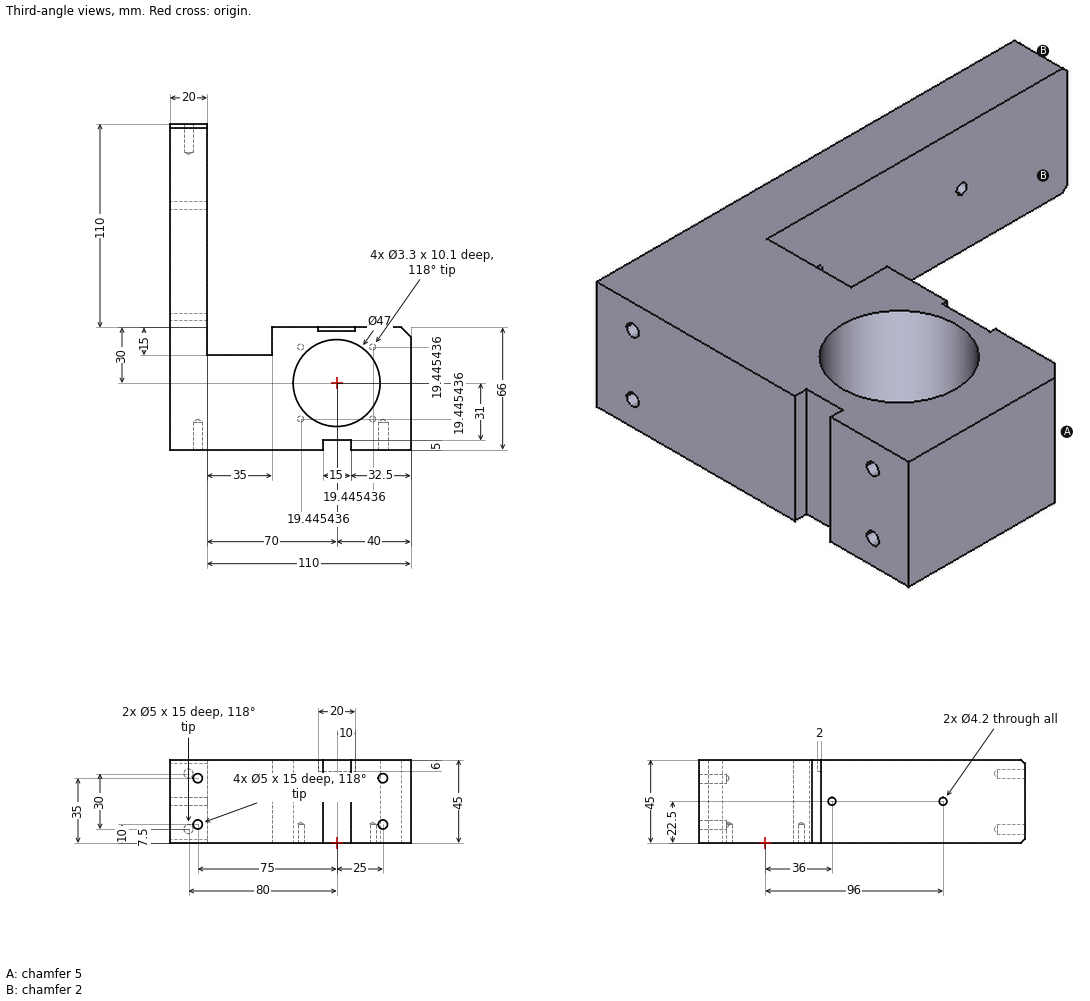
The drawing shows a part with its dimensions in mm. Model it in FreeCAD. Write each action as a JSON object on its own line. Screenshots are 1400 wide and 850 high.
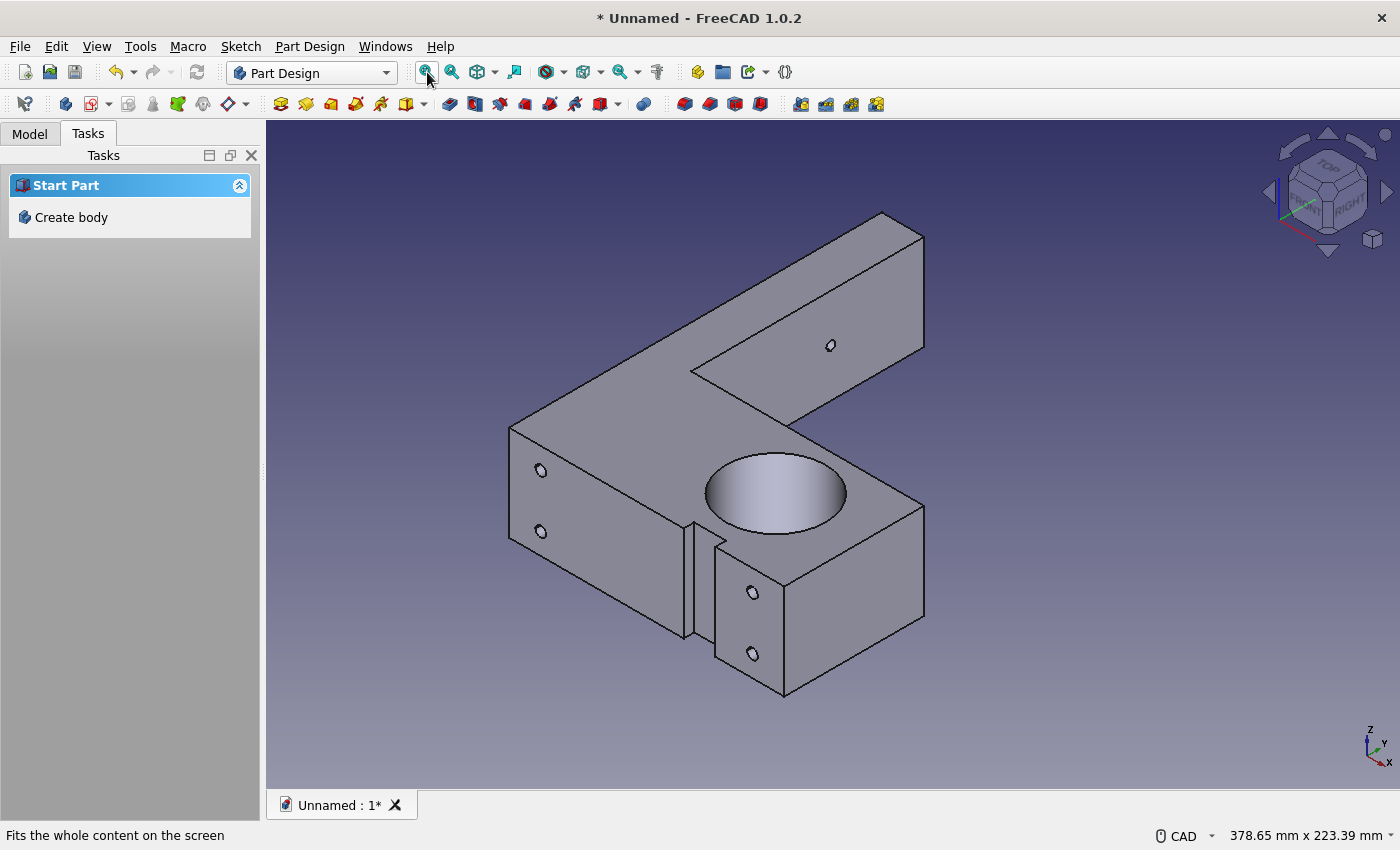
{"action": "key", "text": "2"}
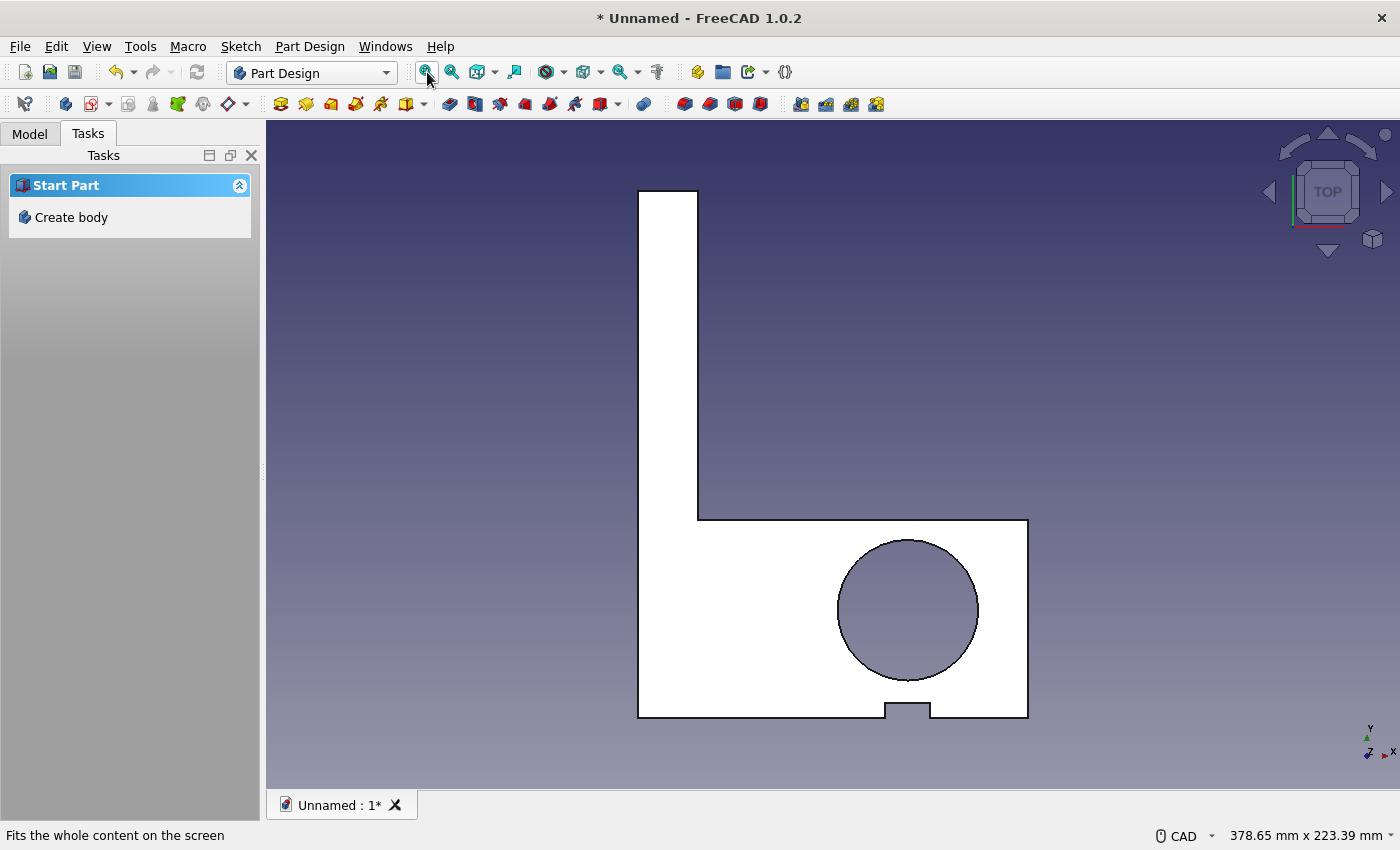
{"action": "key", "text": "1"}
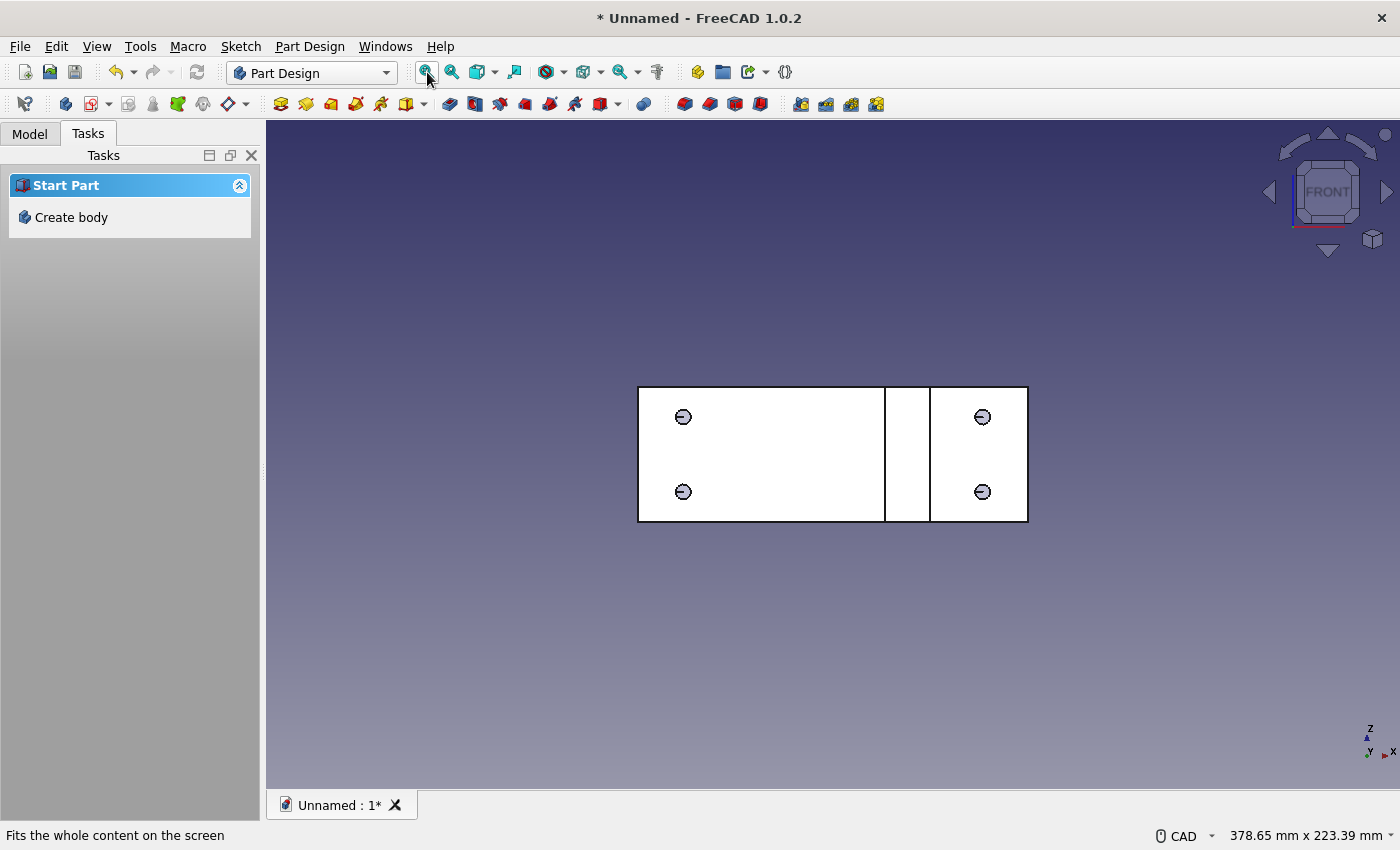
{"action": "left_click", "coordinate": [427, 72]}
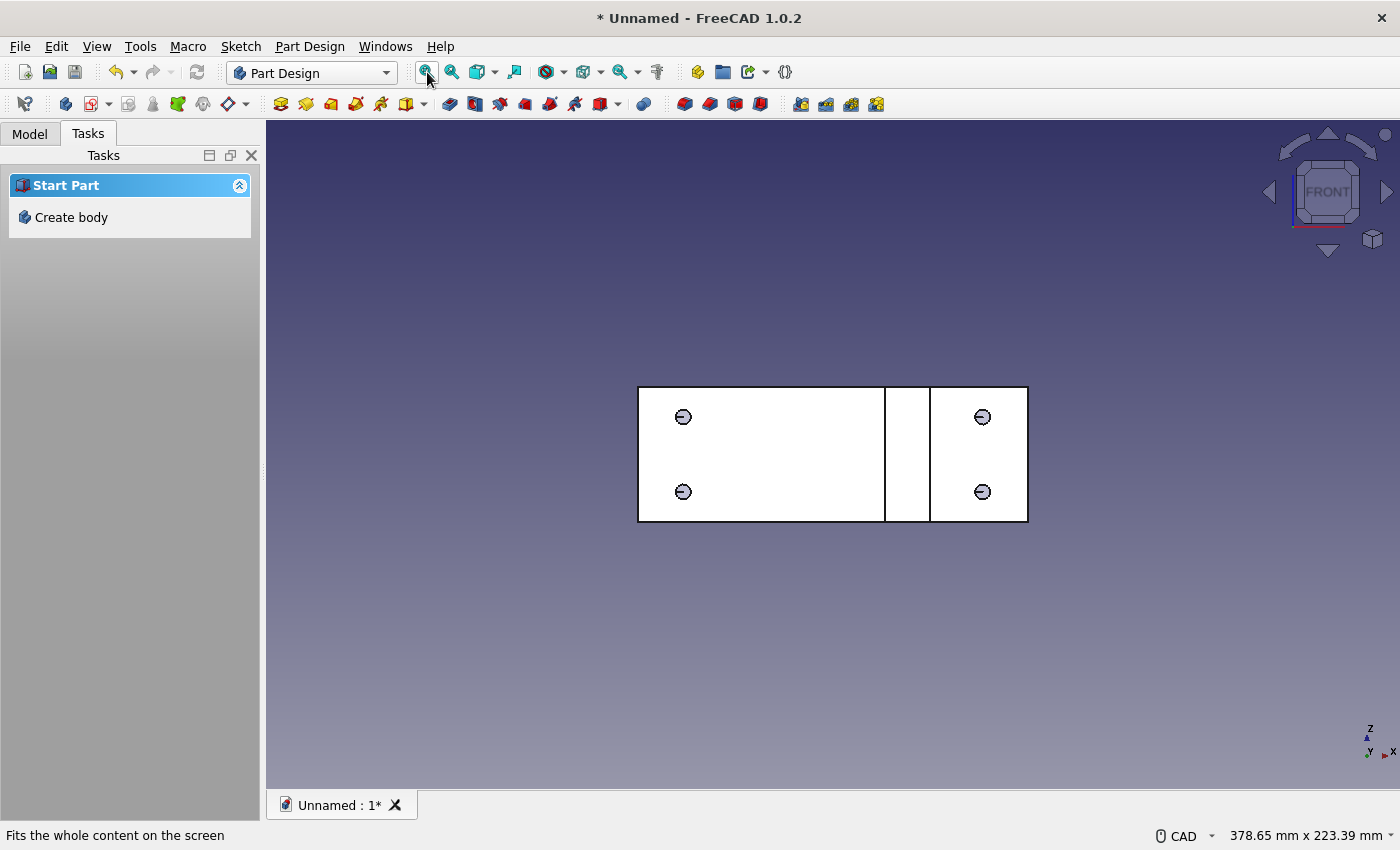
{"action": "key", "text": "3"}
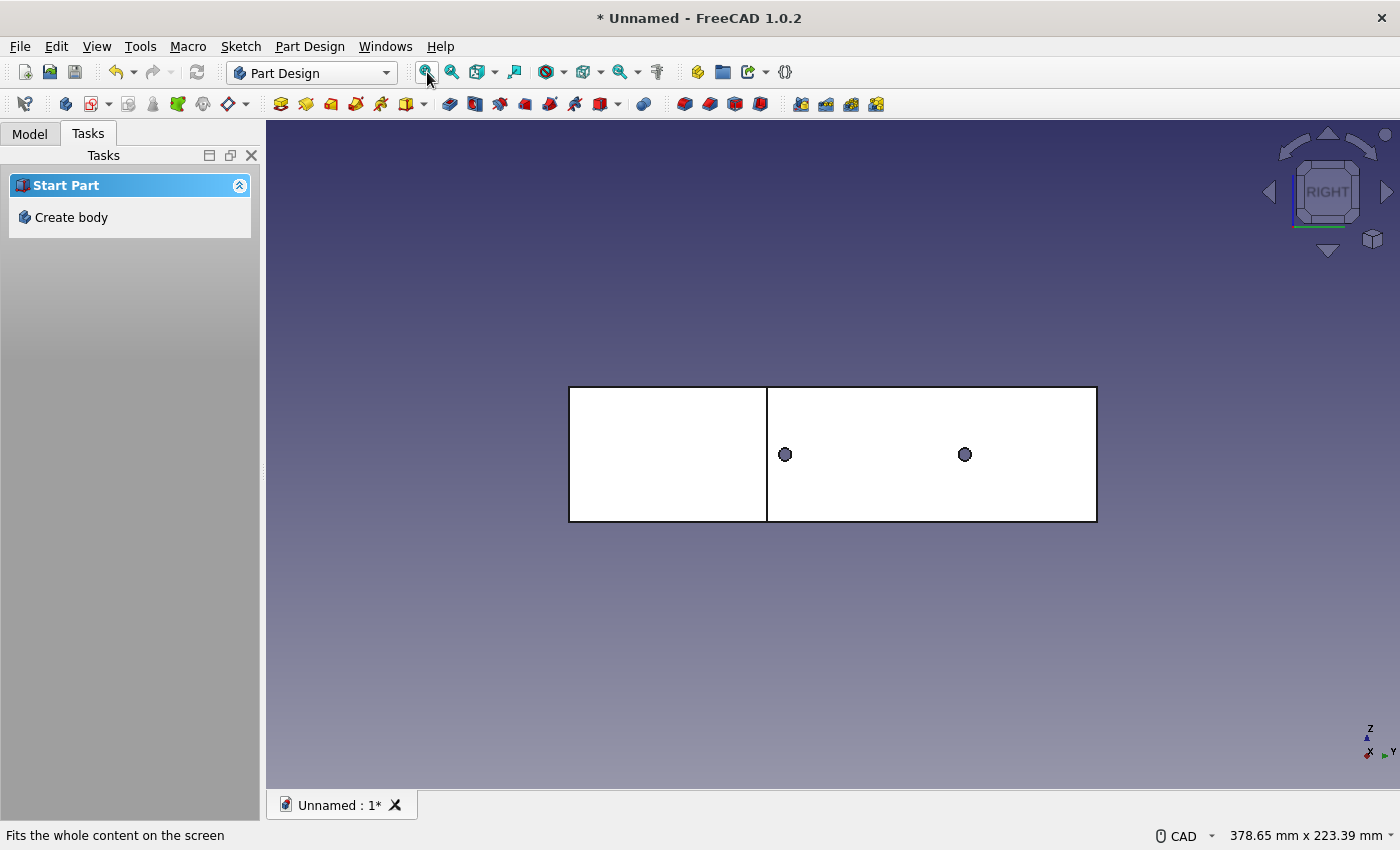
{"action": "left_click", "coordinate": [767, 453]}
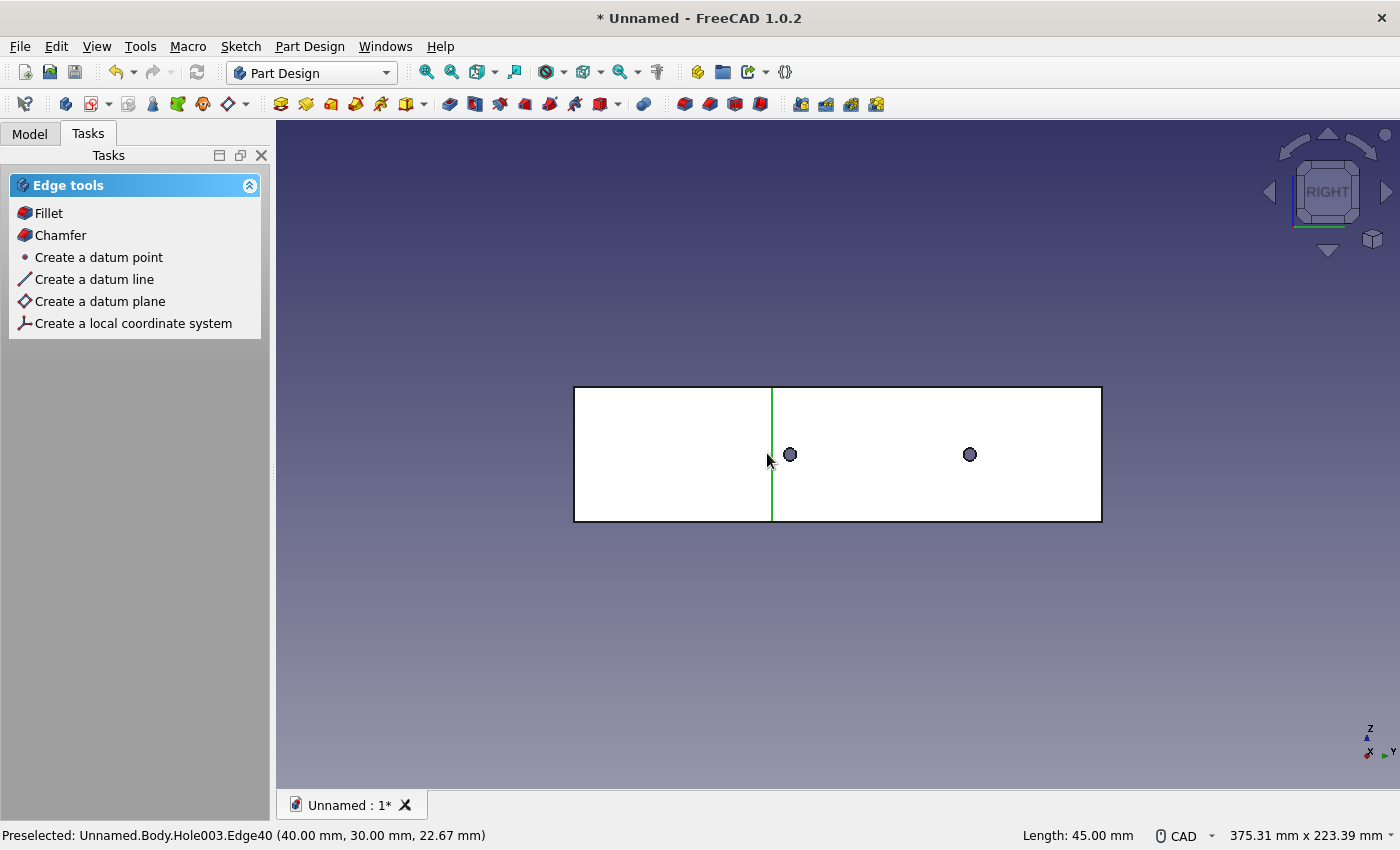
{"action": "left_click", "coordinate": [710, 104]}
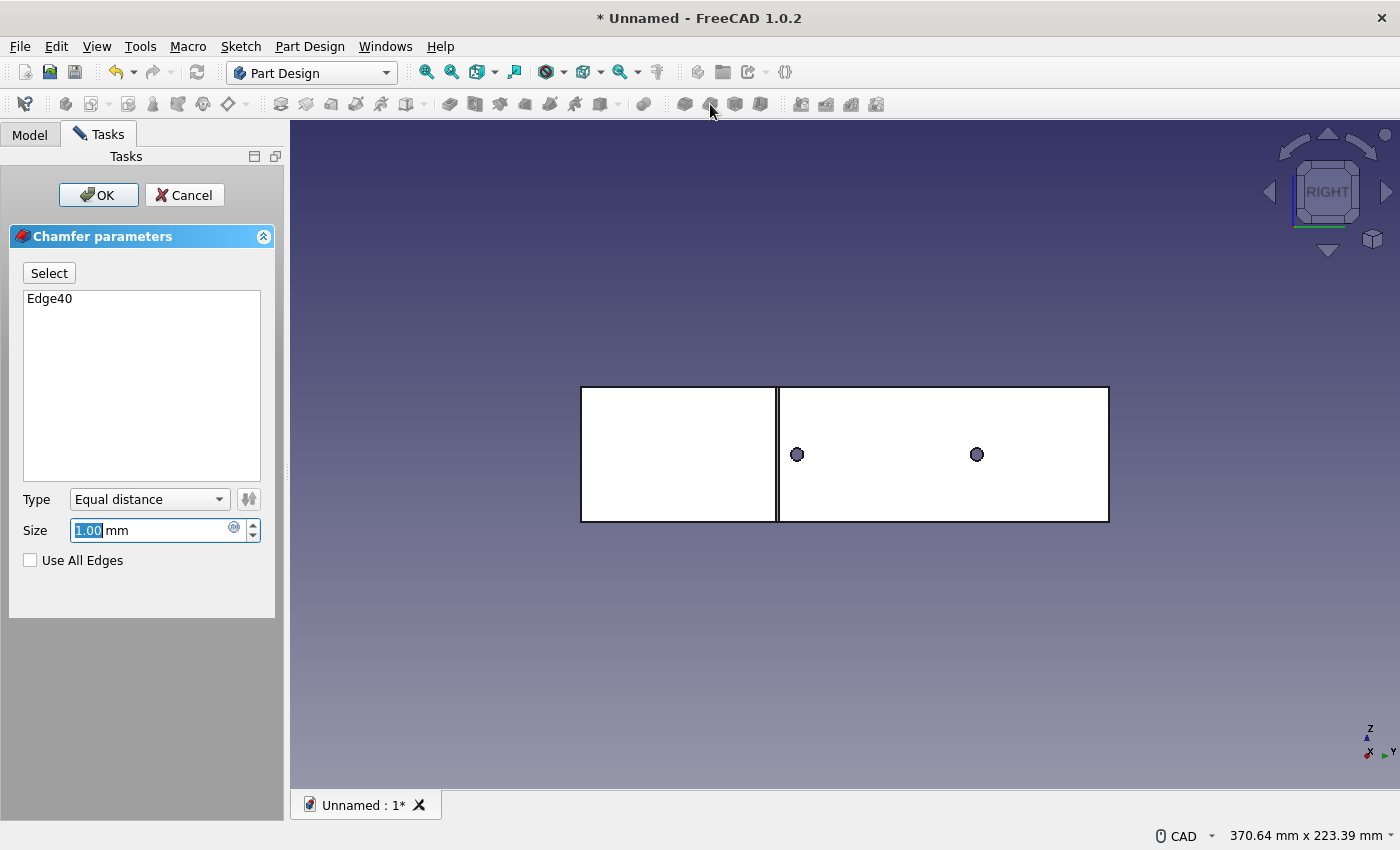
{"action": "type", "text": "5"}
{"action": "key", "text": "Tab"}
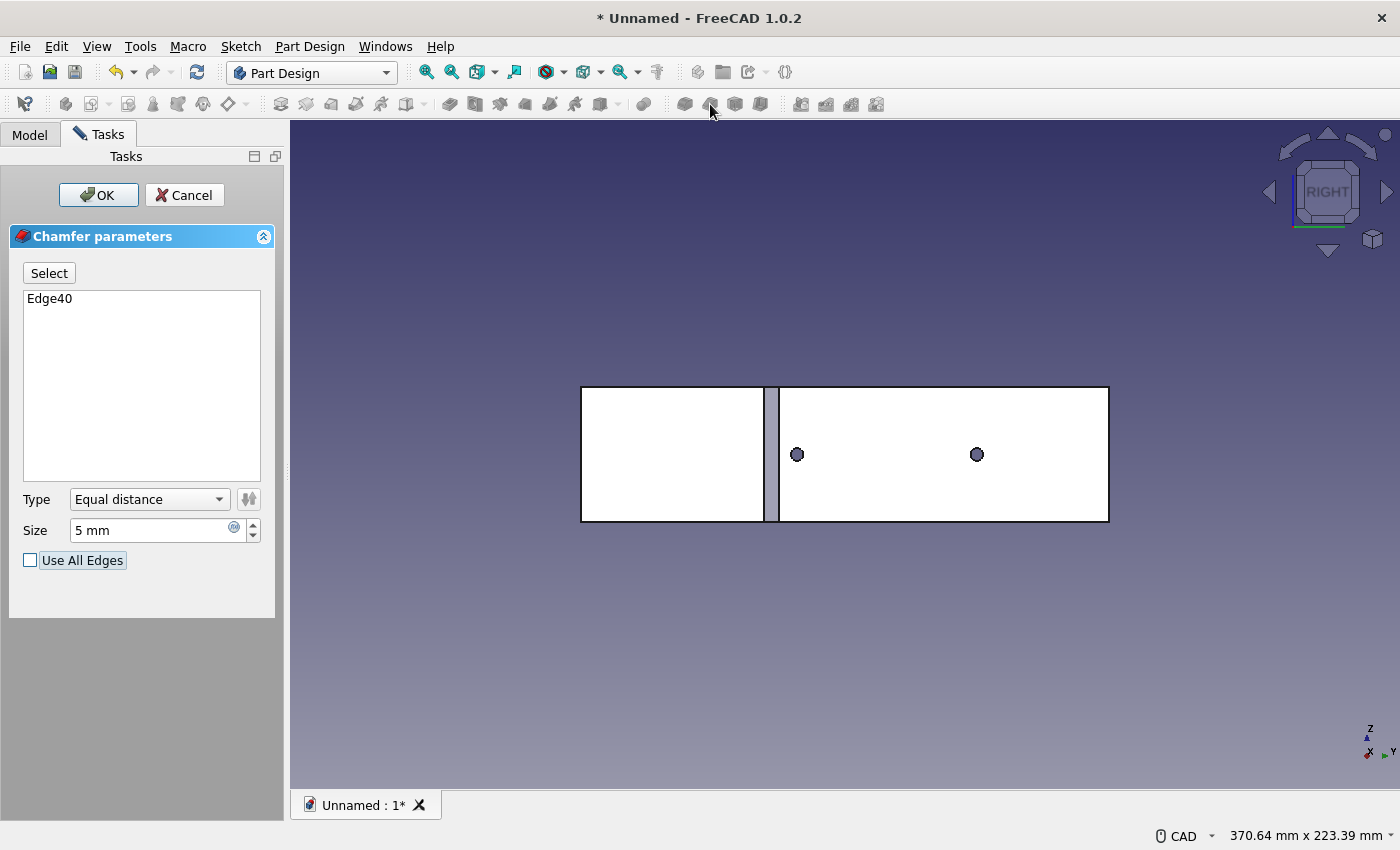
{"action": "left_click", "coordinate": [99, 195]}